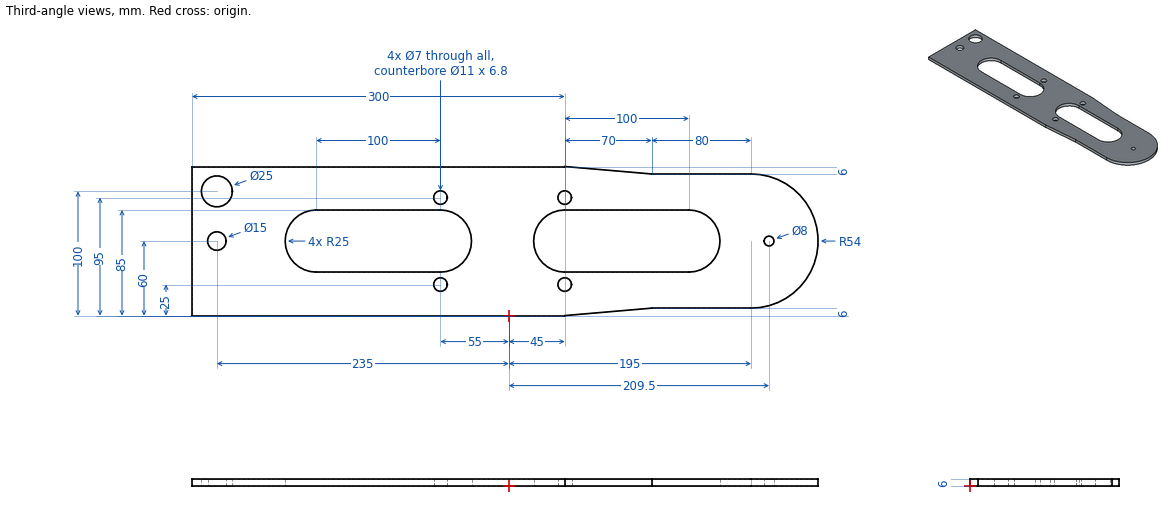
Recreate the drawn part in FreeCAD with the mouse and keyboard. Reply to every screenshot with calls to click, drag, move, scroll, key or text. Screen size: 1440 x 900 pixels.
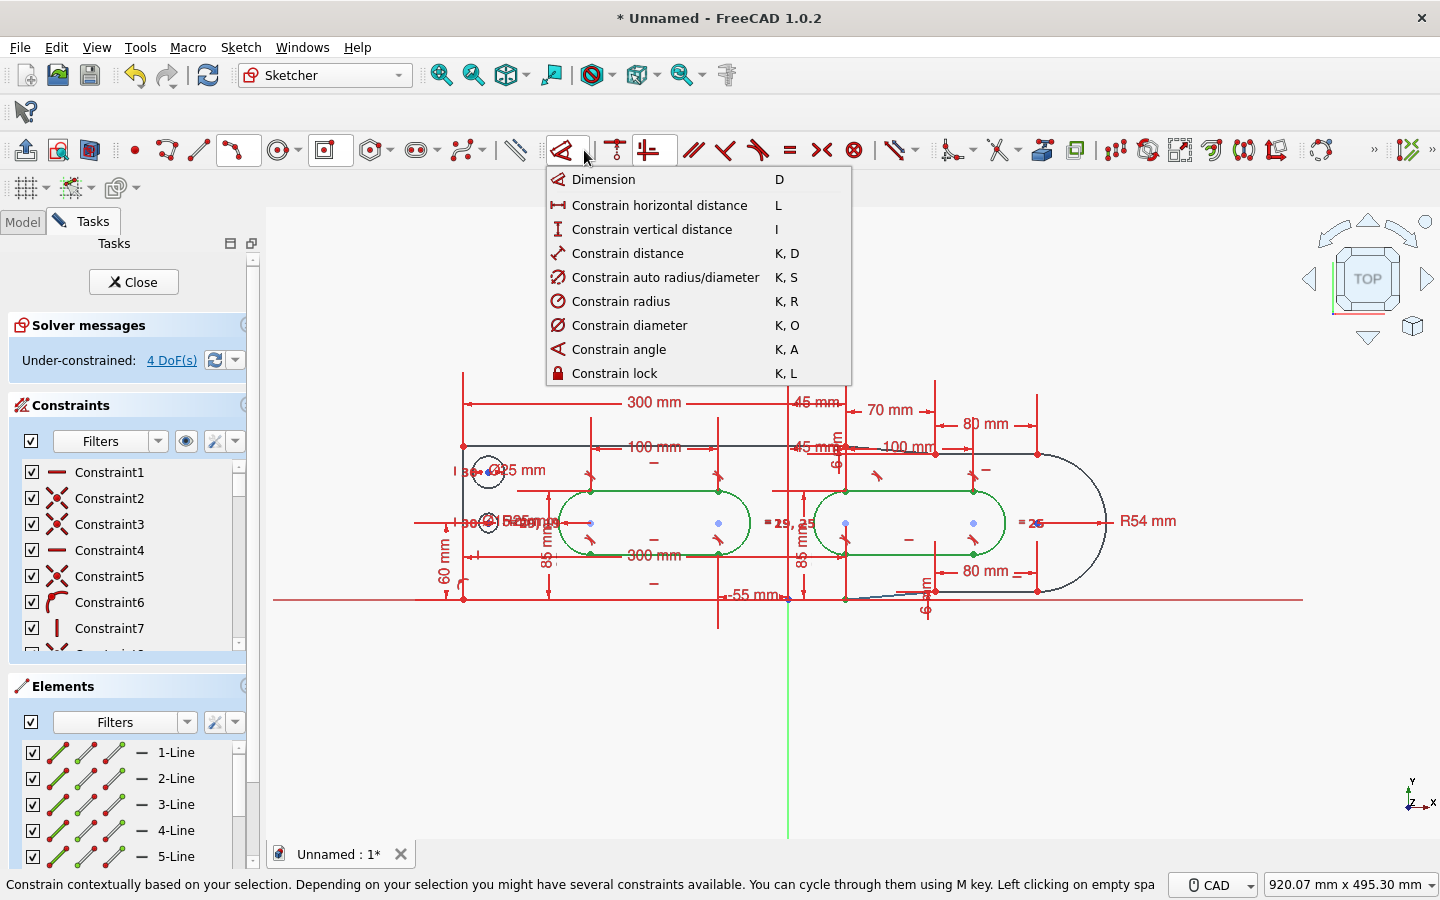
click(699, 205)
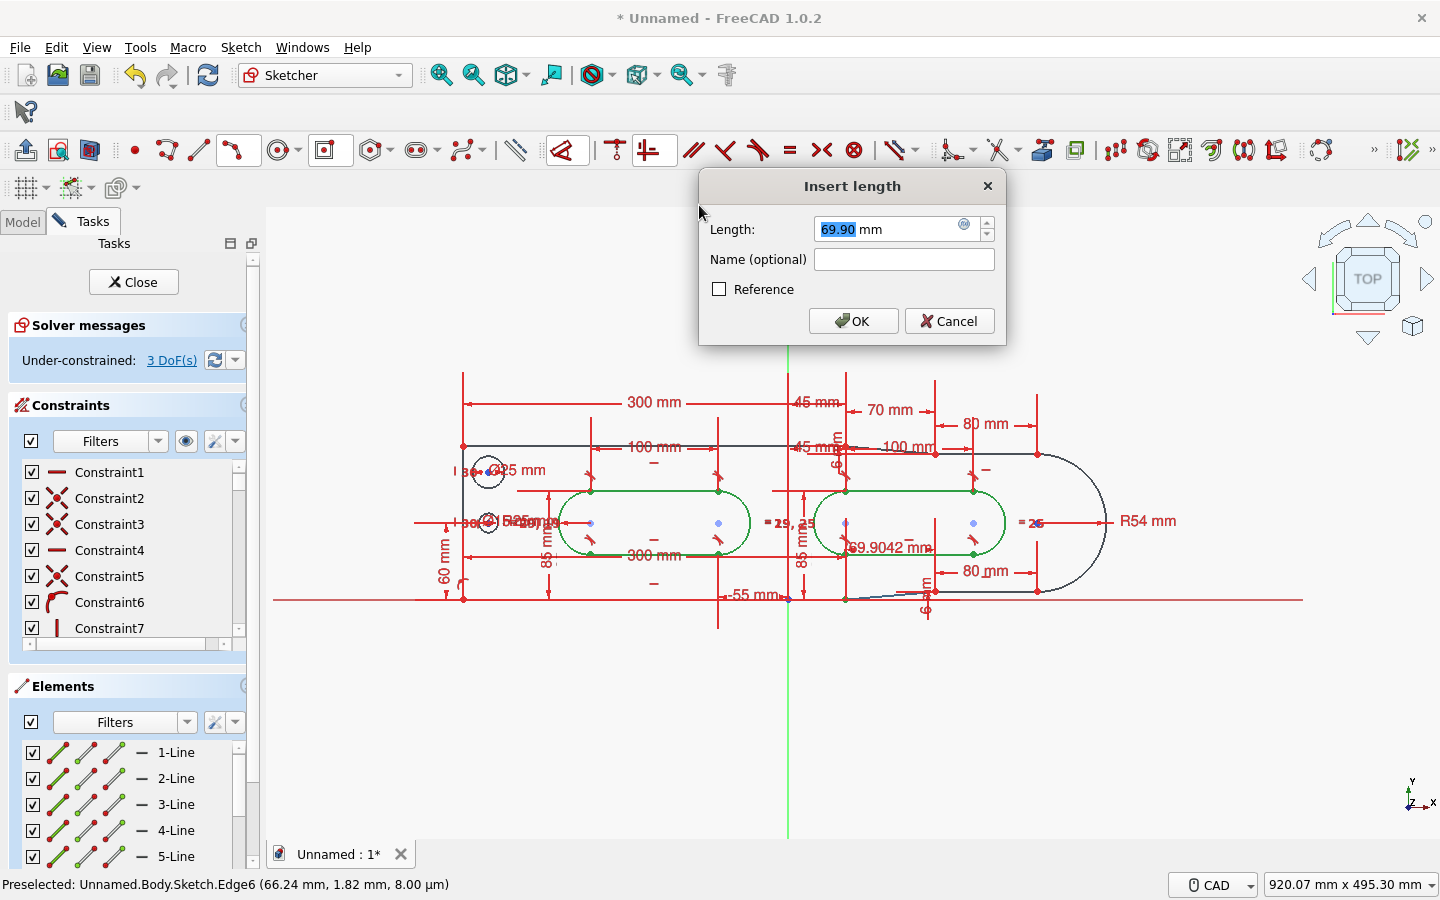
text(70)
key(Return)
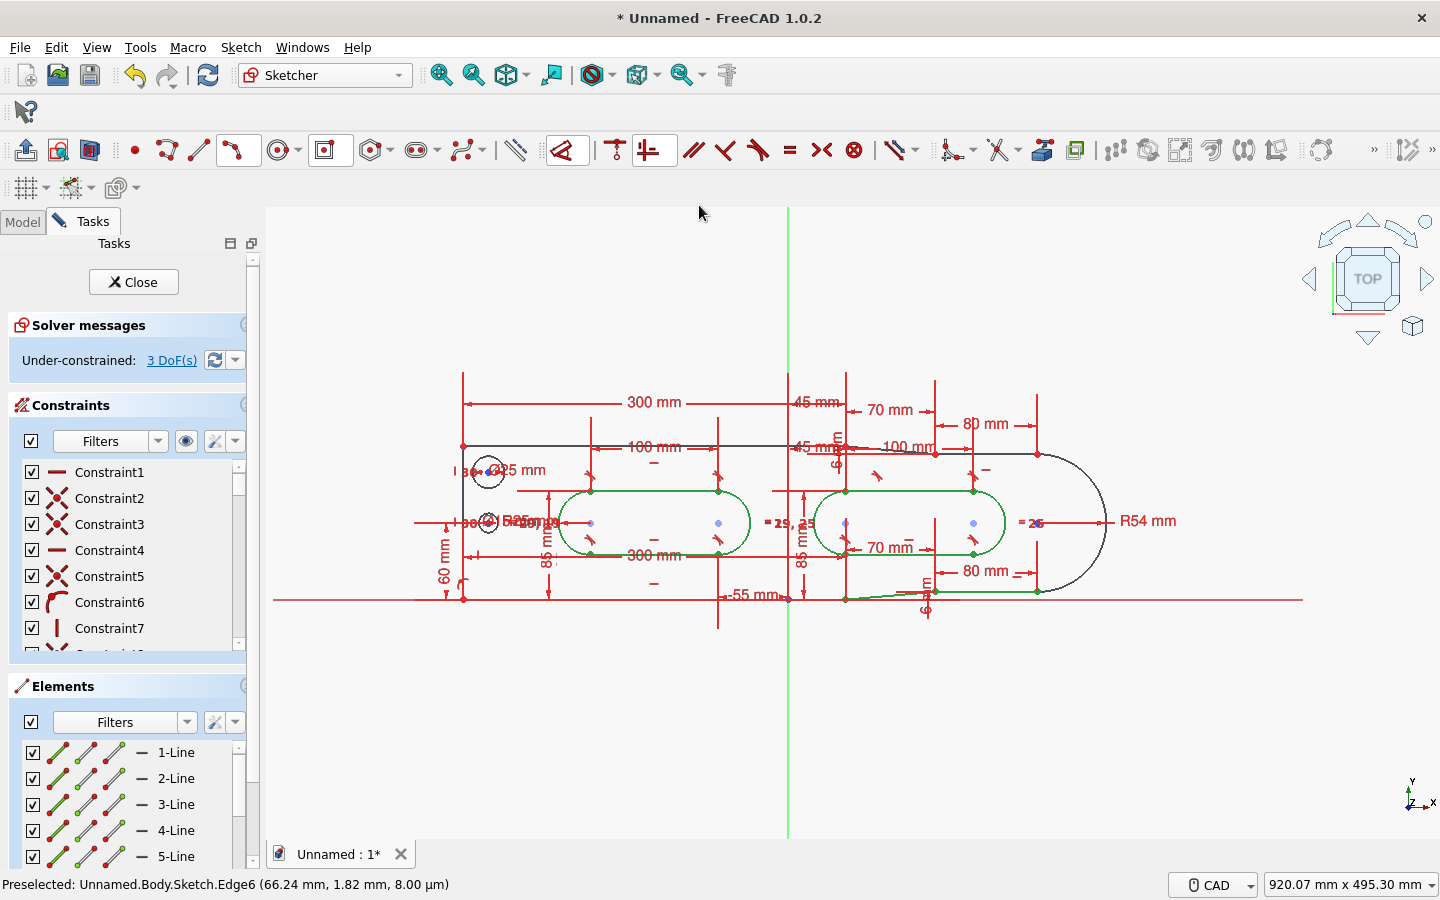
click(488, 523)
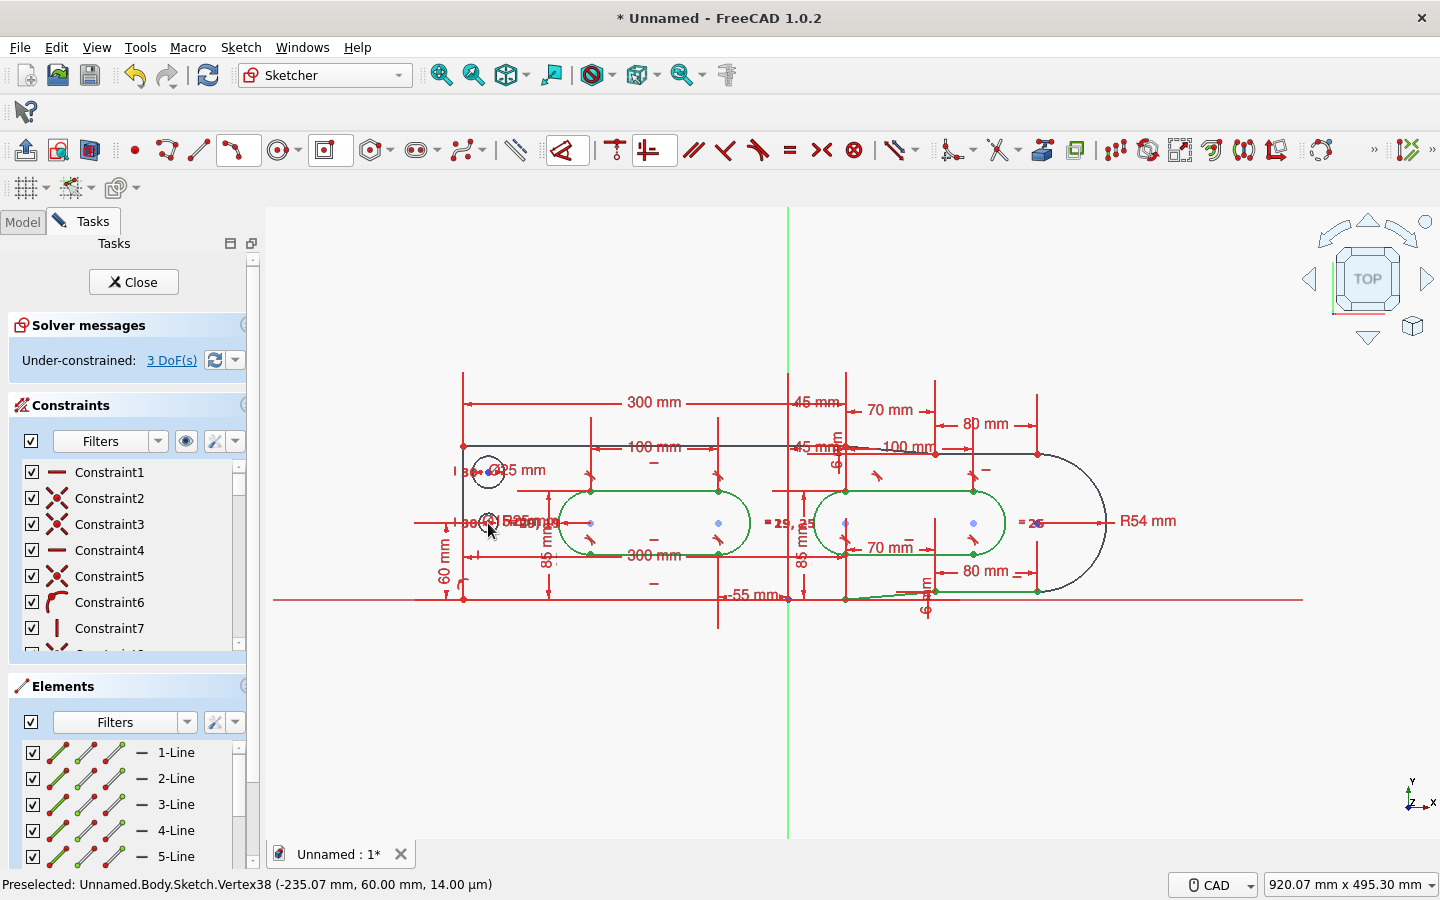
click(584, 150)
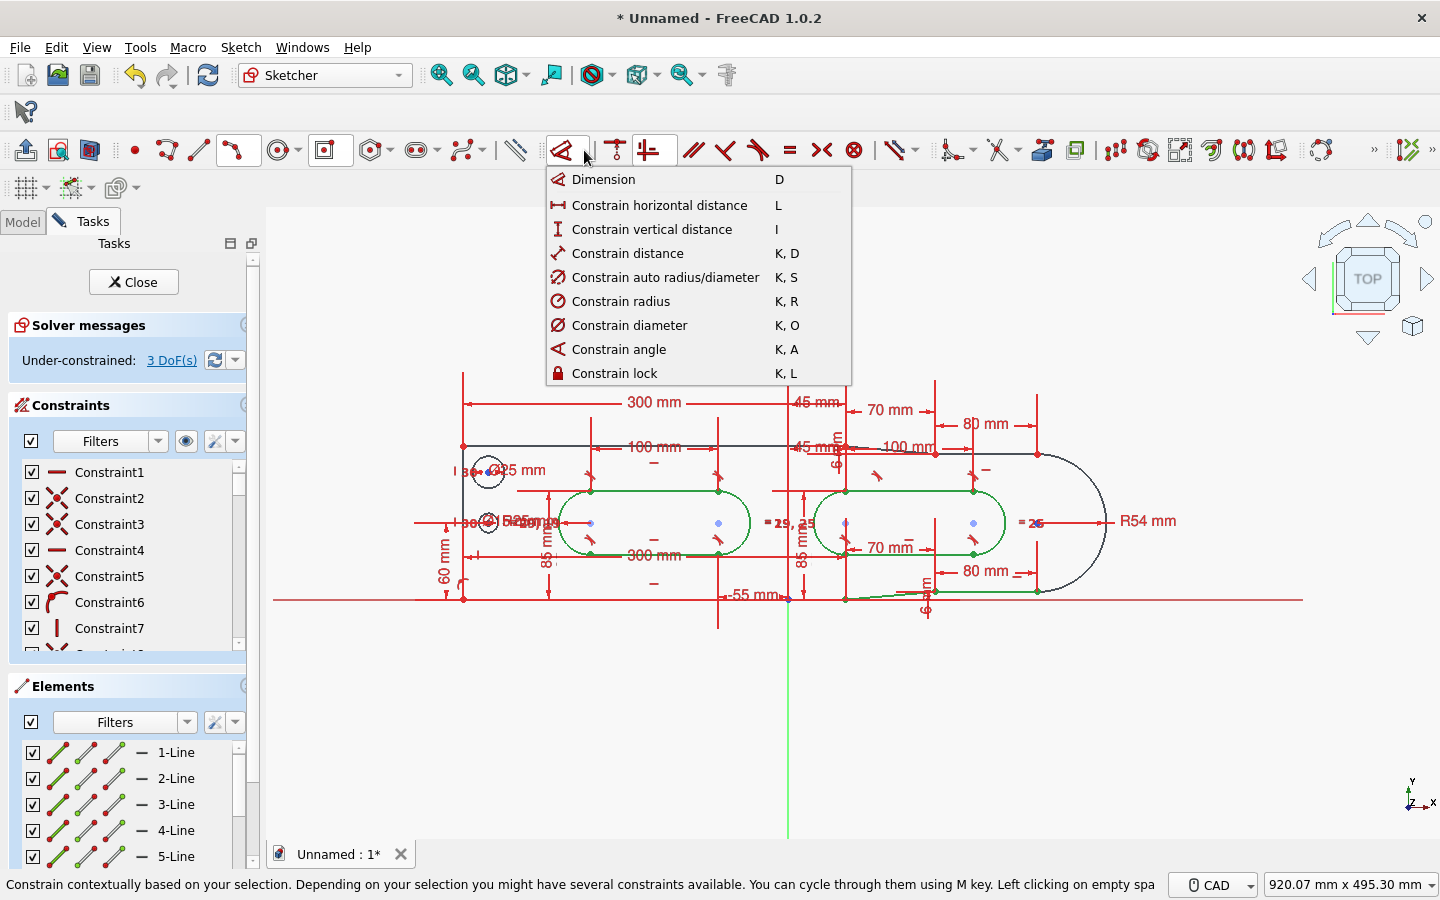
click(699, 205)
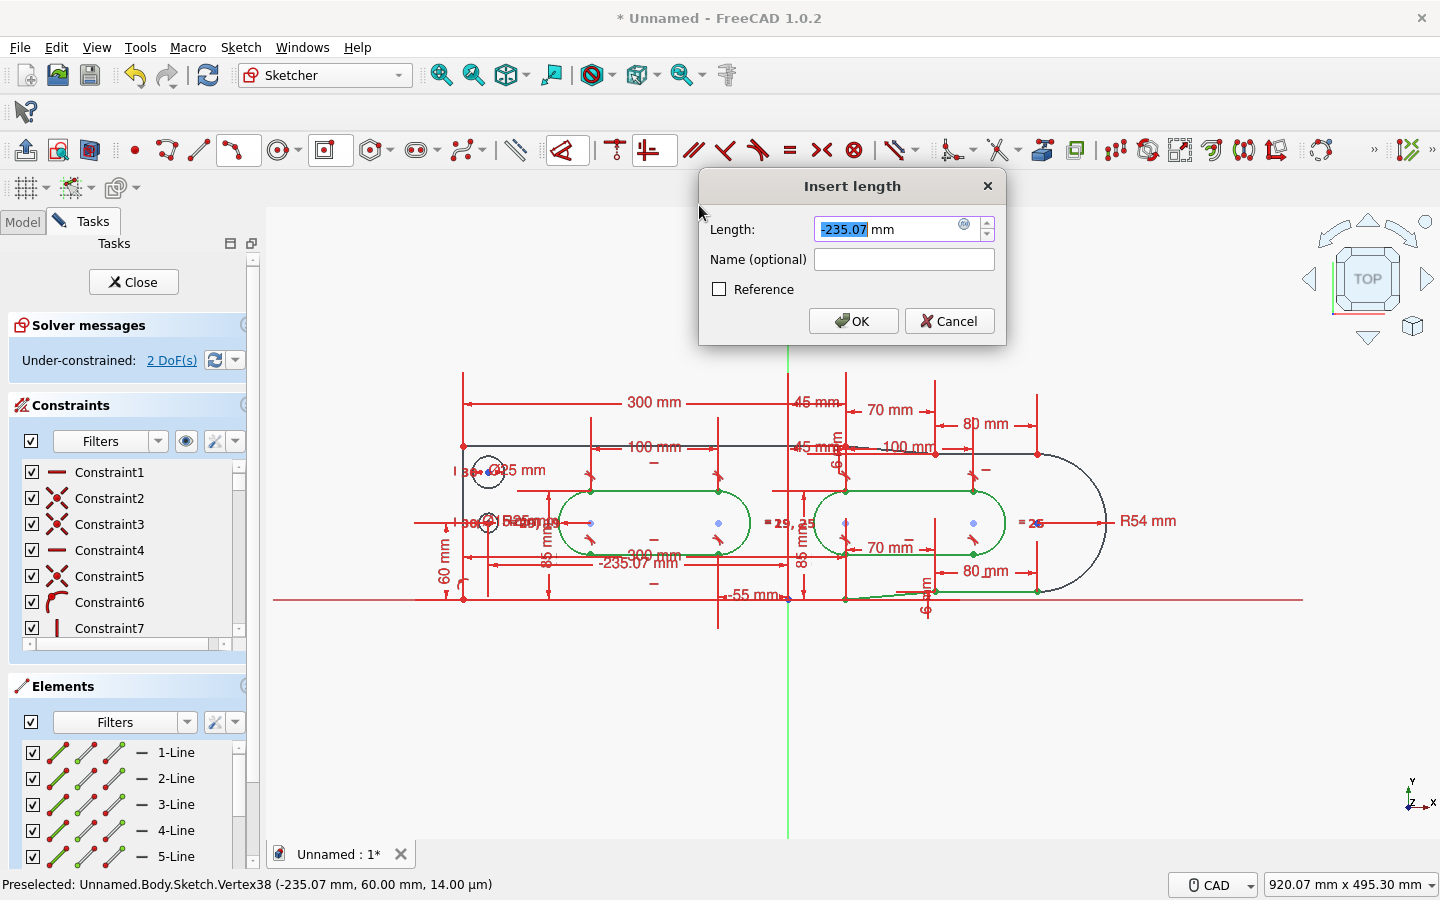
text(-235)
key(Return)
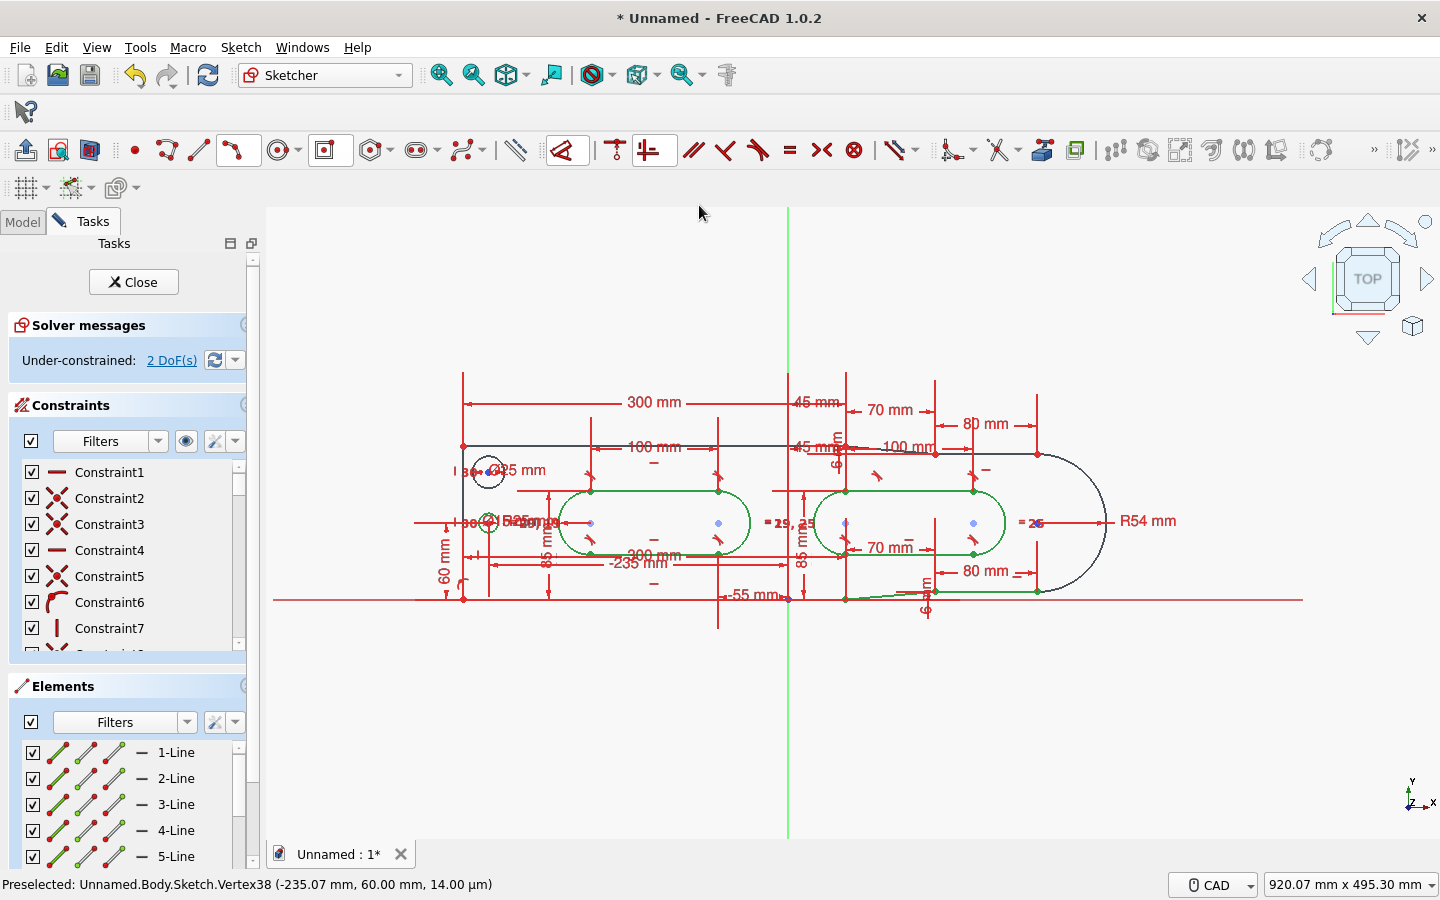
click(489, 472)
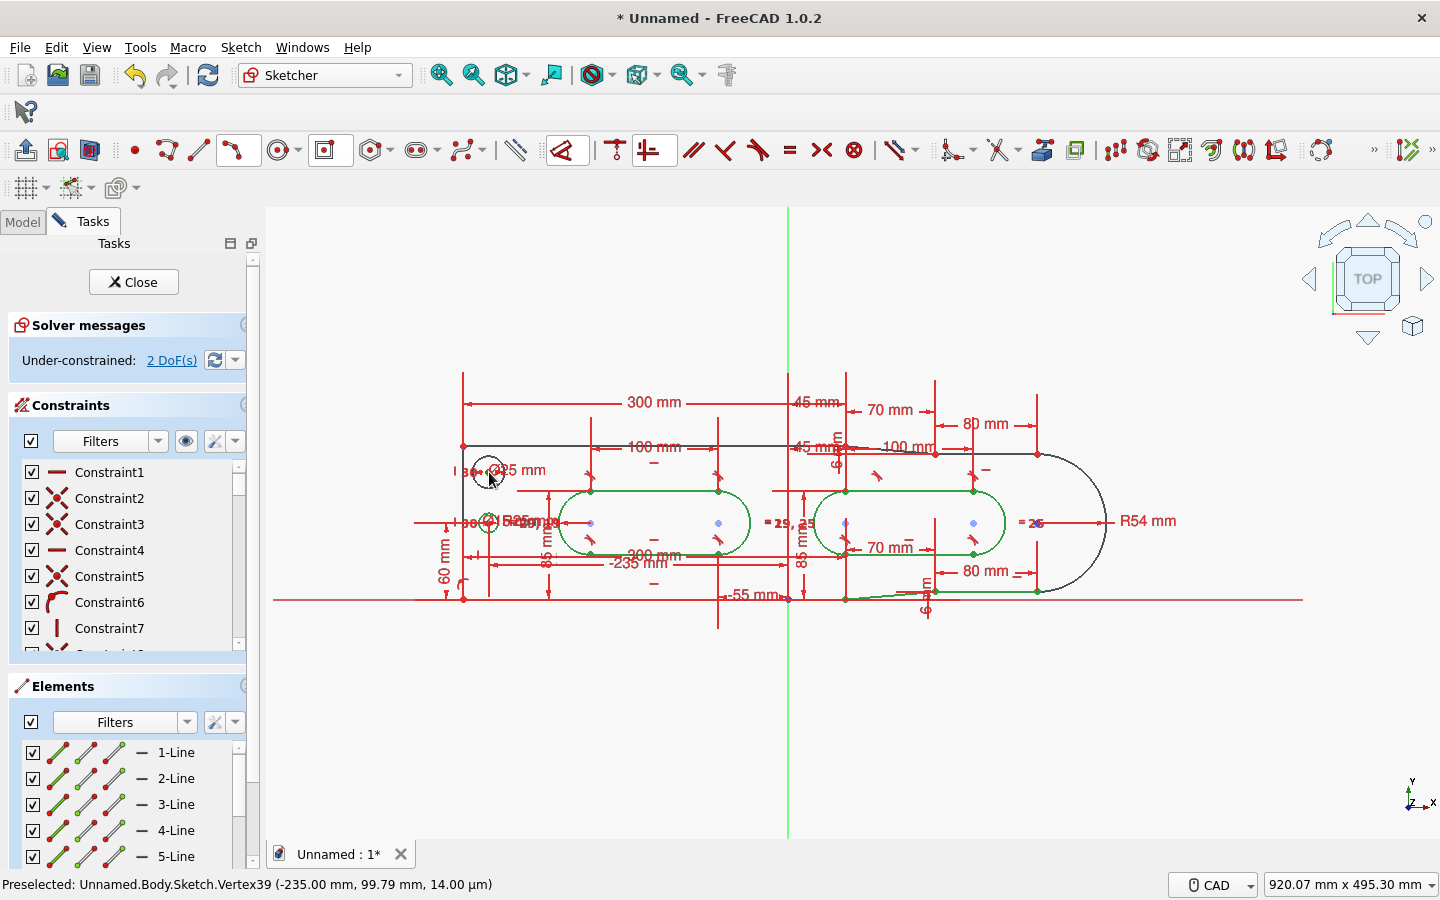
key(i)